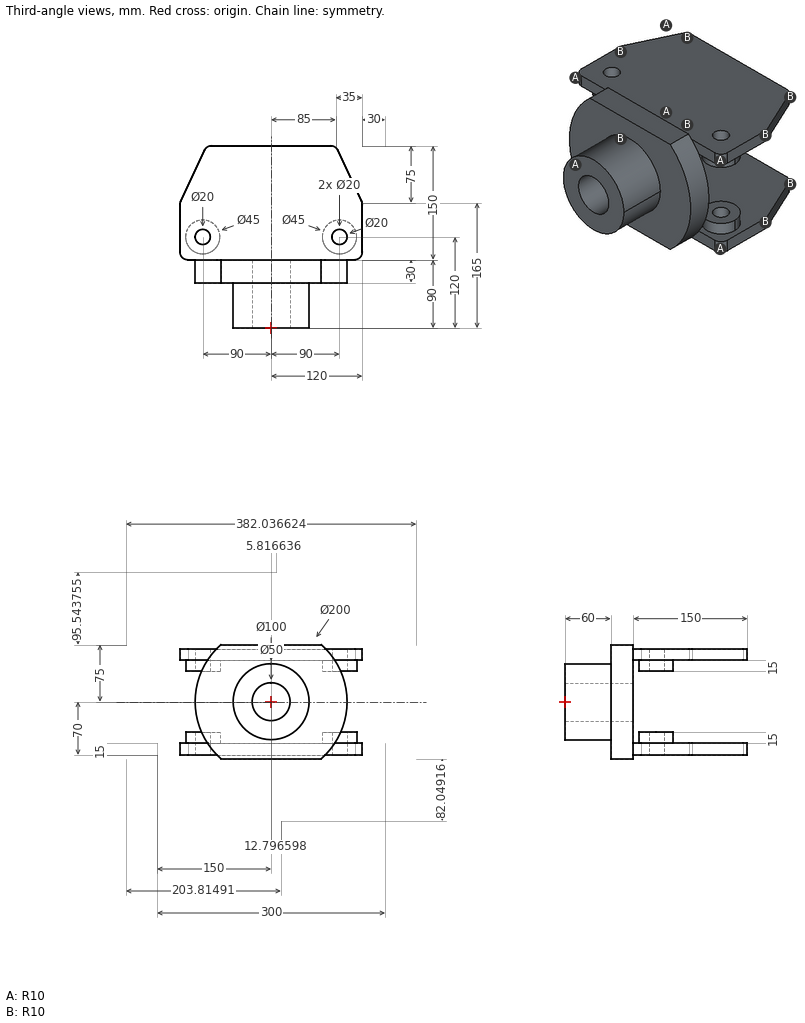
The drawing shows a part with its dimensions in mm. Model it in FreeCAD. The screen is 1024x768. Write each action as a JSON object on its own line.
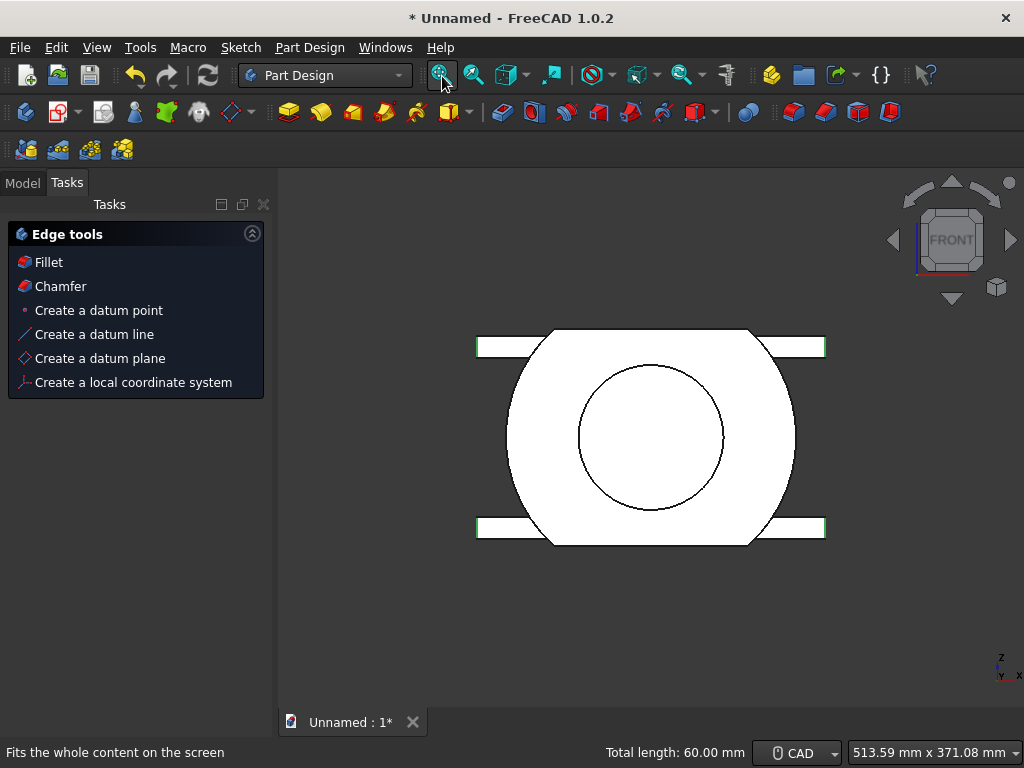
{"action": "left_click", "coordinate": [825, 346], "text": "ctrl"}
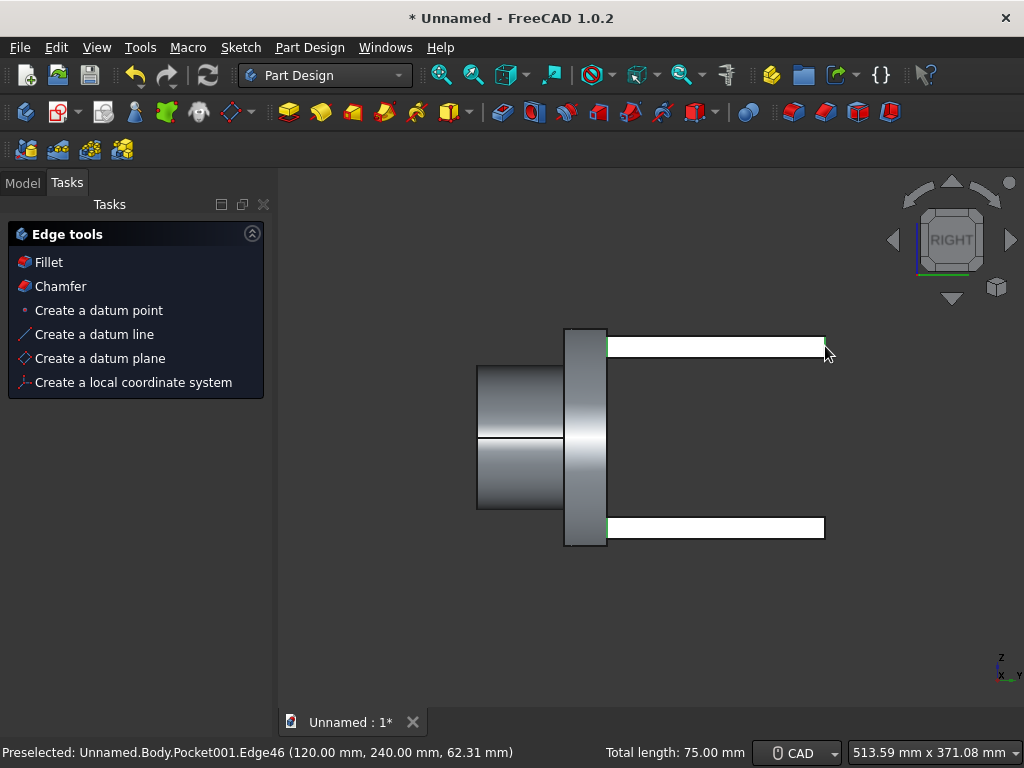
{"action": "left_click", "coordinate": [825, 527], "text": "ctrl"}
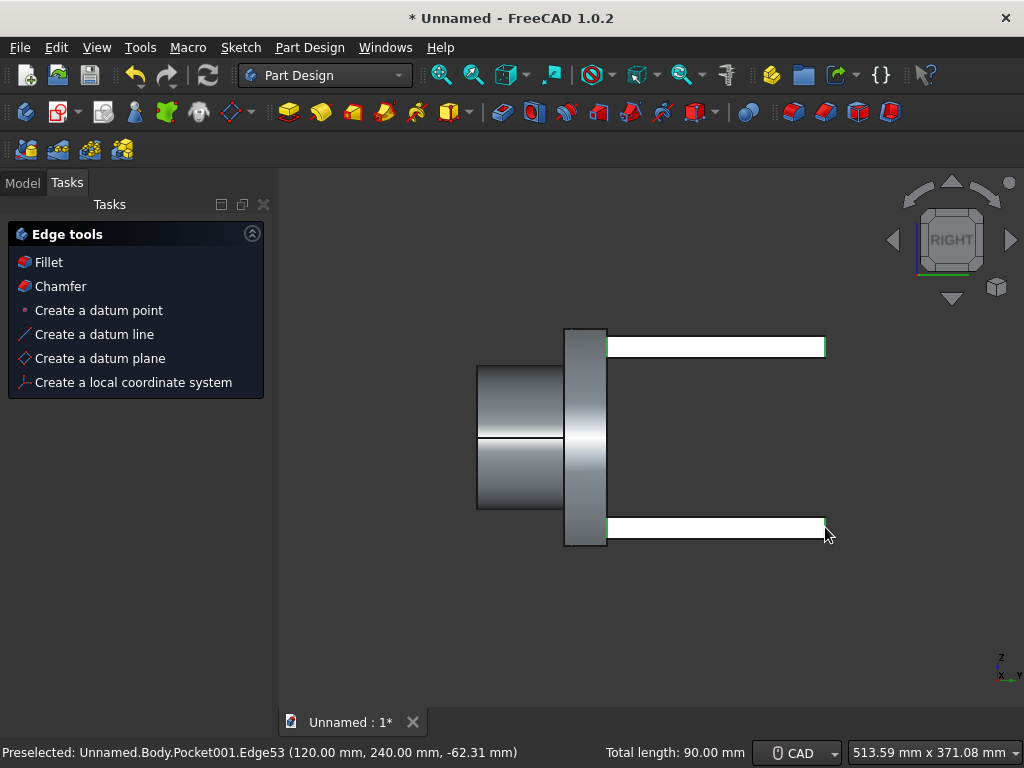
{"action": "scroll", "coordinate": [825, 527], "scroll_direction": "up", "scroll_amount": 4}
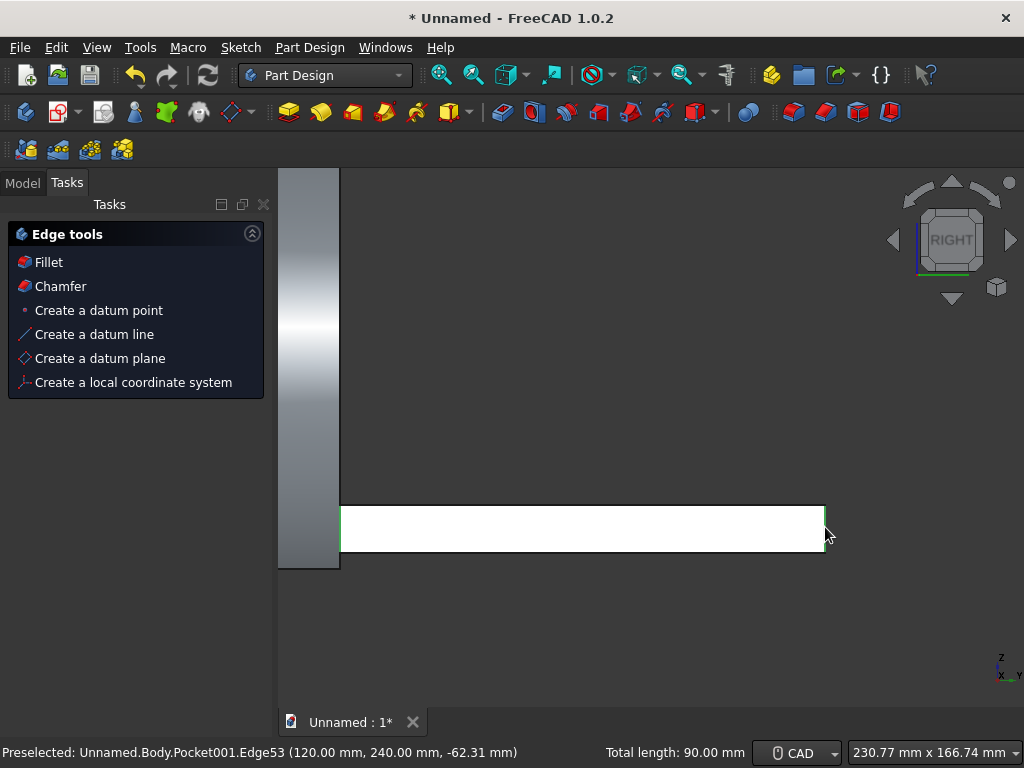
{"action": "left_click", "coordinate": [442, 76]}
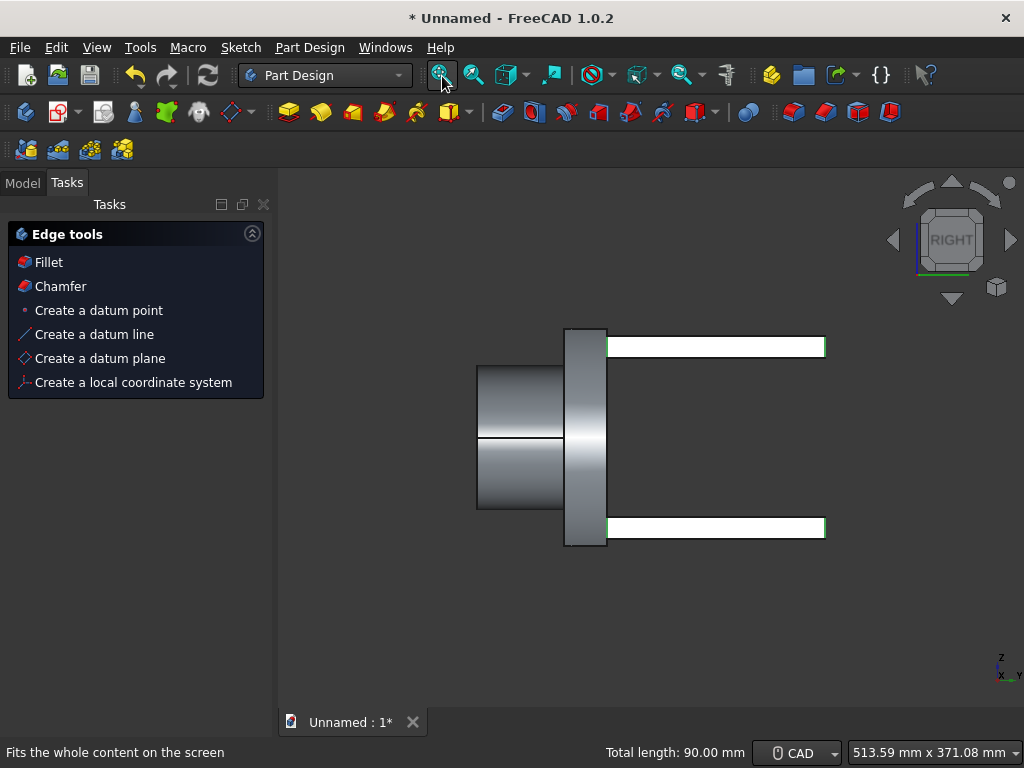
{"action": "key", "text": "5"}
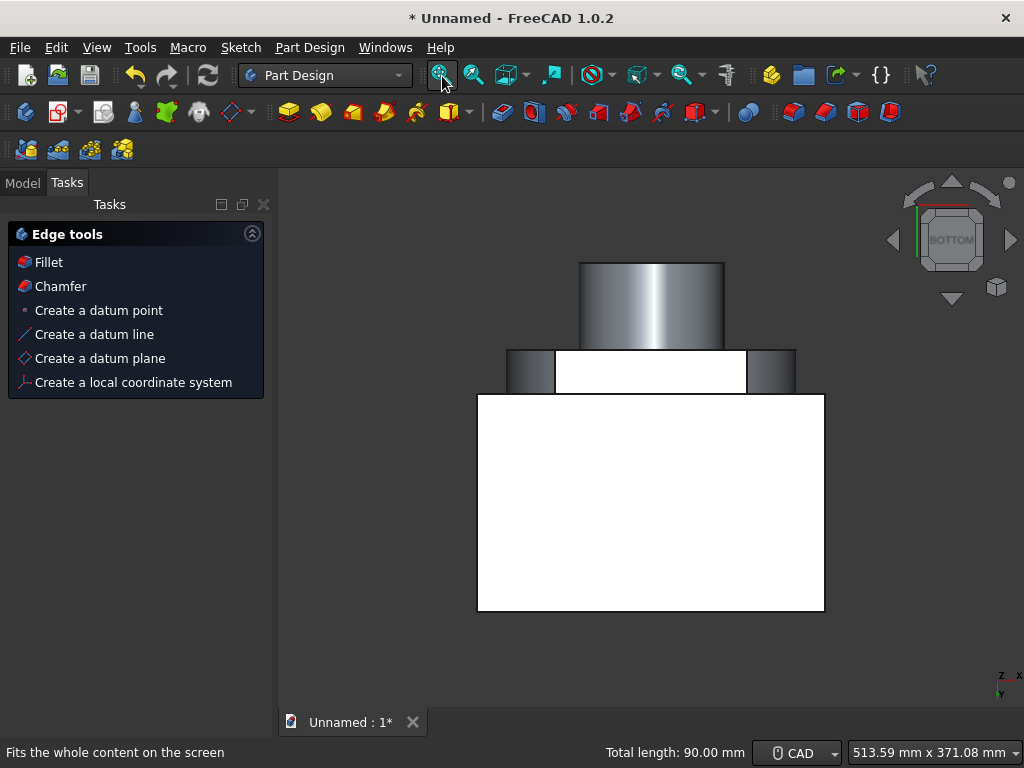
{"action": "scroll", "coordinate": [477, 611], "scroll_direction": "up", "scroll_amount": 4}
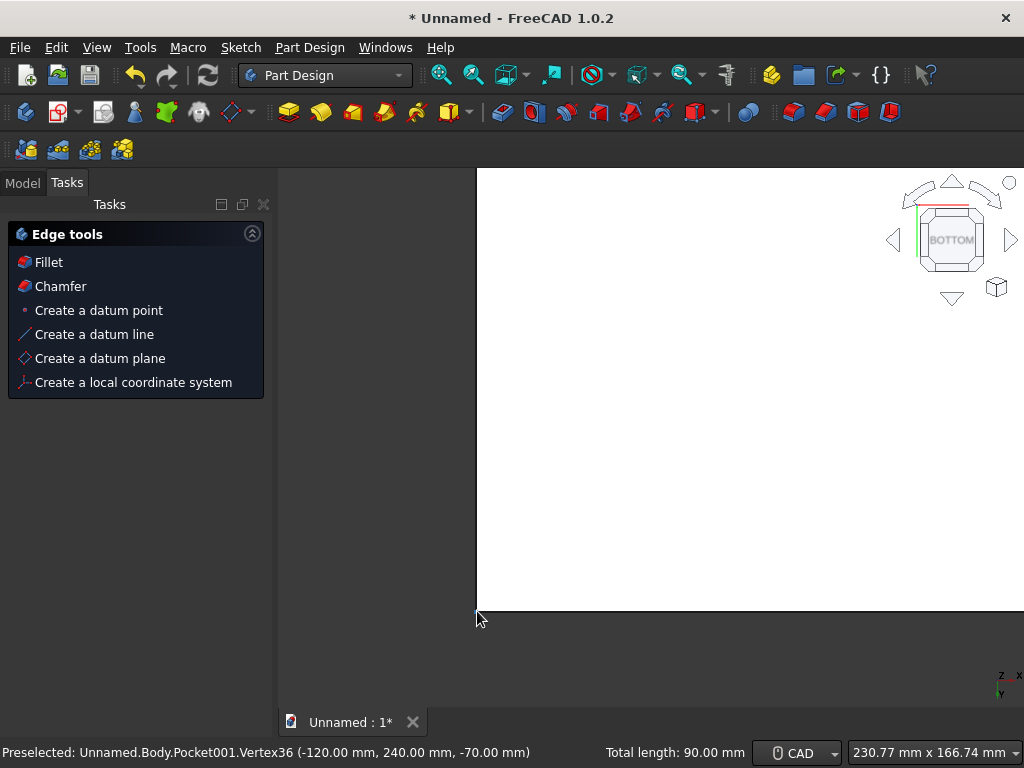
{"action": "left_click", "coordinate": [442, 76]}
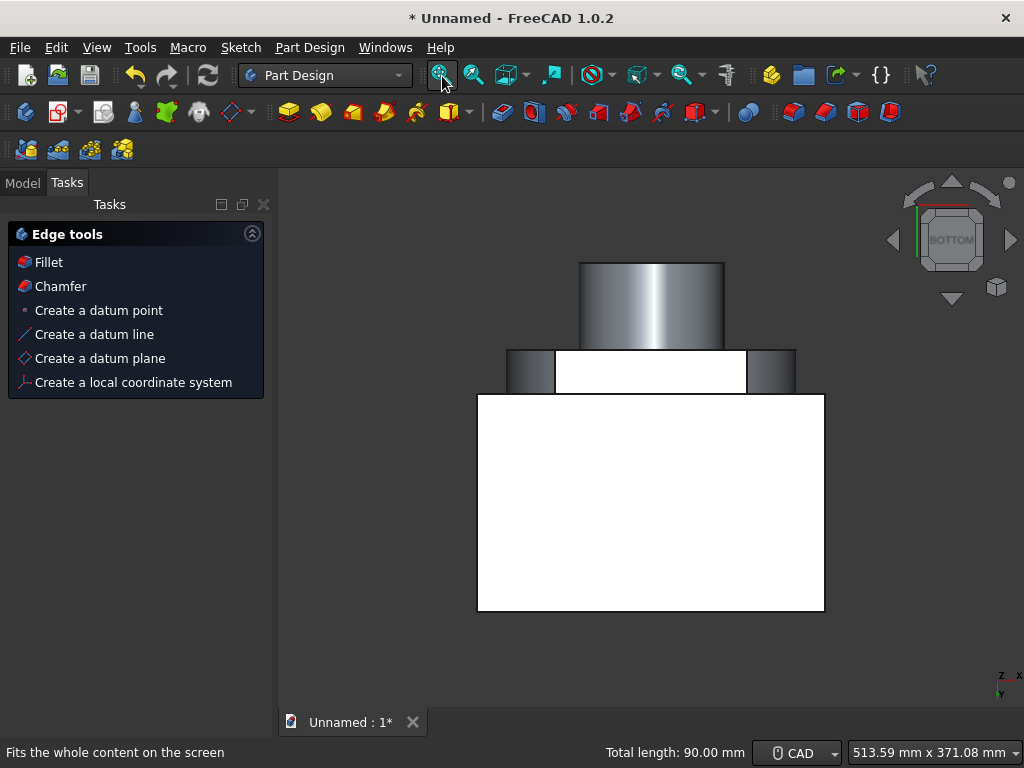
{"action": "key", "text": "4"}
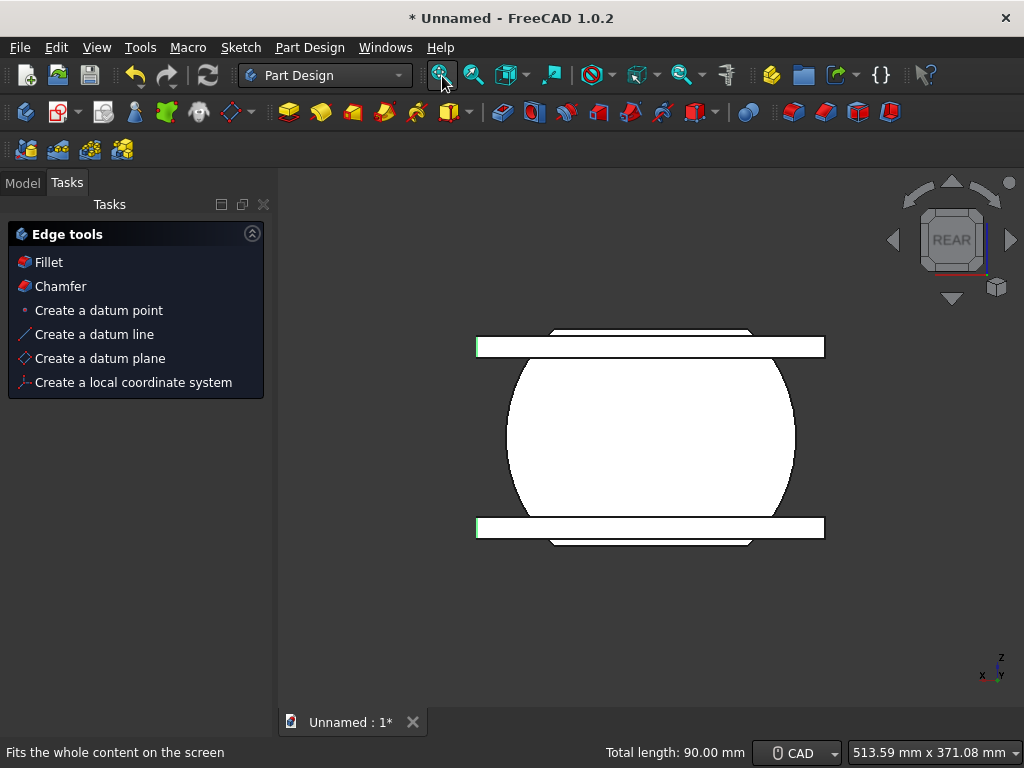
{"action": "left_click", "coordinate": [825, 527], "text": "ctrl"}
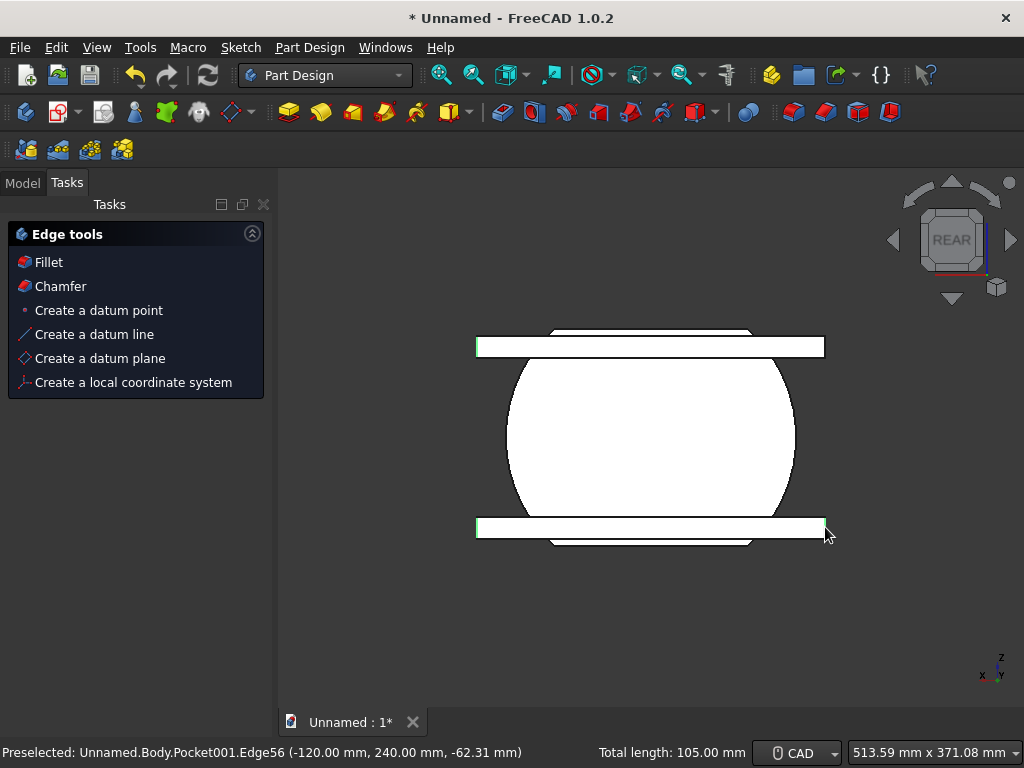
{"action": "left_click", "coordinate": [825, 346], "text": "ctrl"}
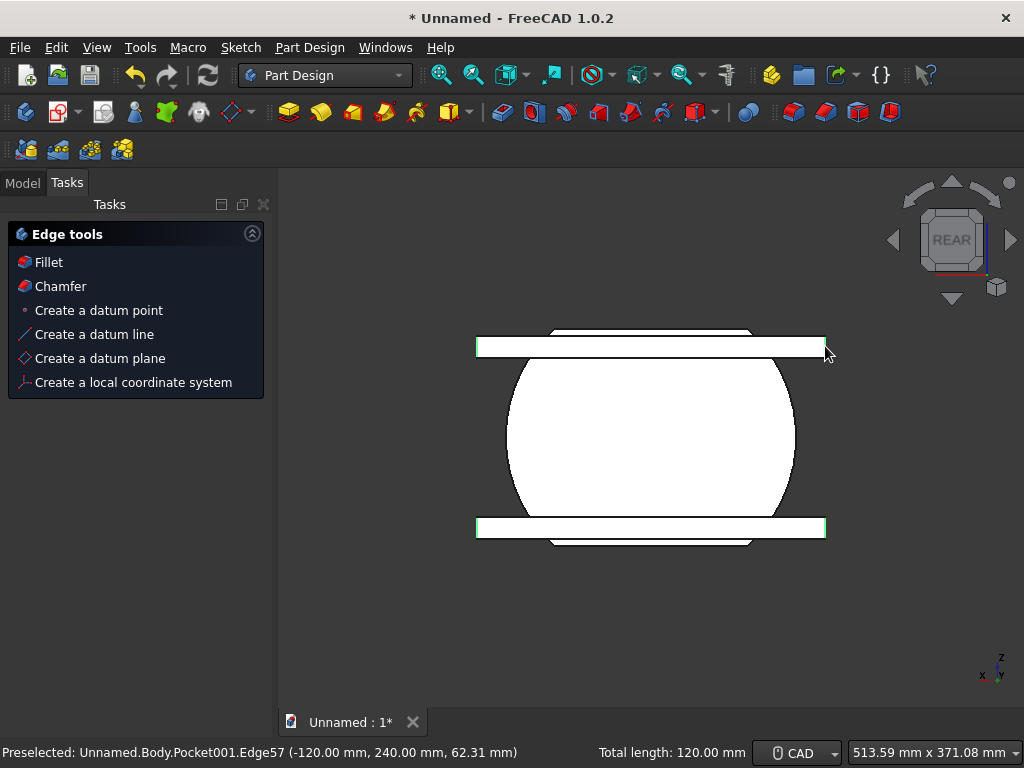
{"action": "left_click", "coordinate": [794, 112]}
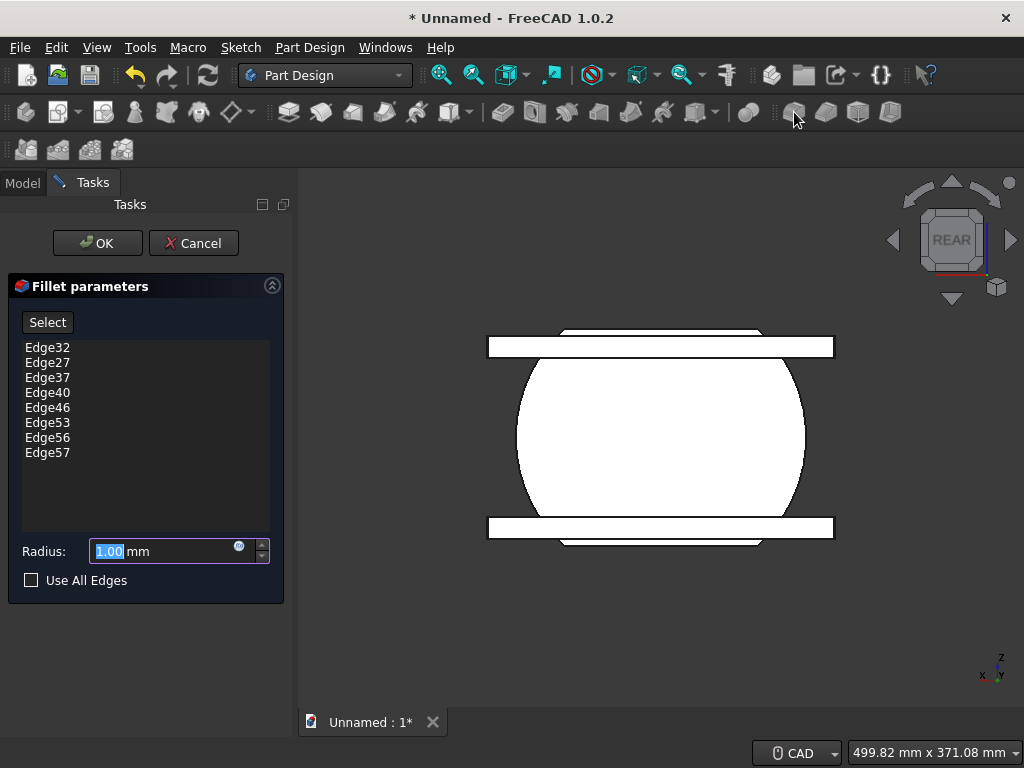
{"action": "type", "text": "10"}
{"action": "key", "text": "Tab"}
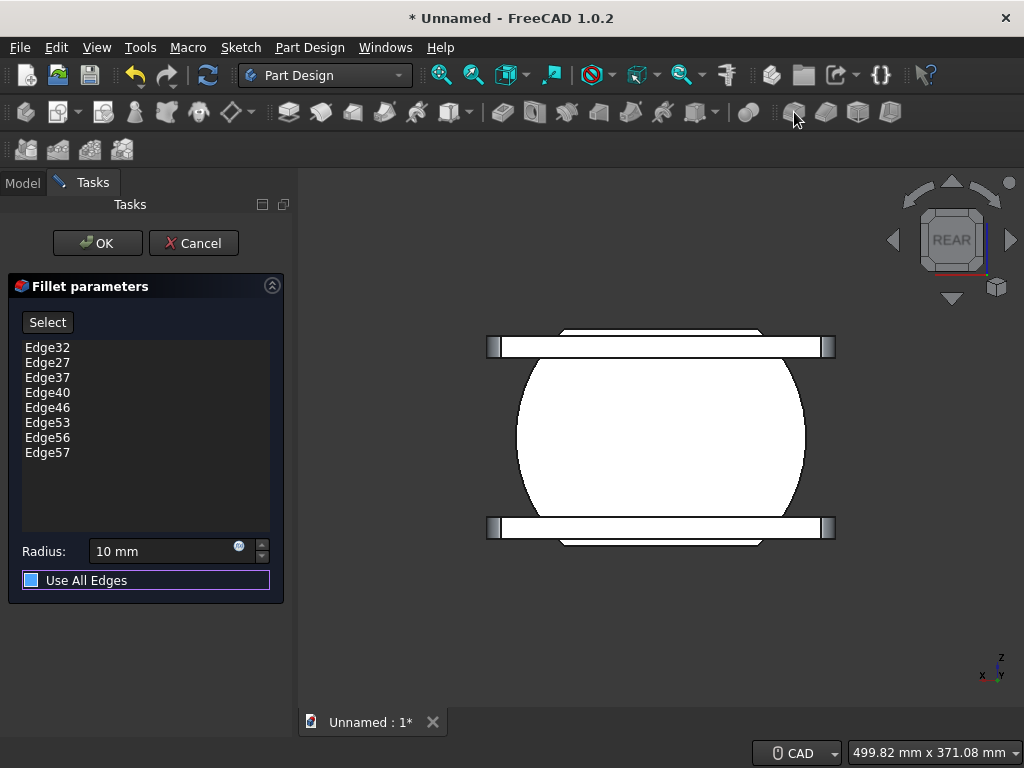
{"action": "left_click", "coordinate": [98, 243]}